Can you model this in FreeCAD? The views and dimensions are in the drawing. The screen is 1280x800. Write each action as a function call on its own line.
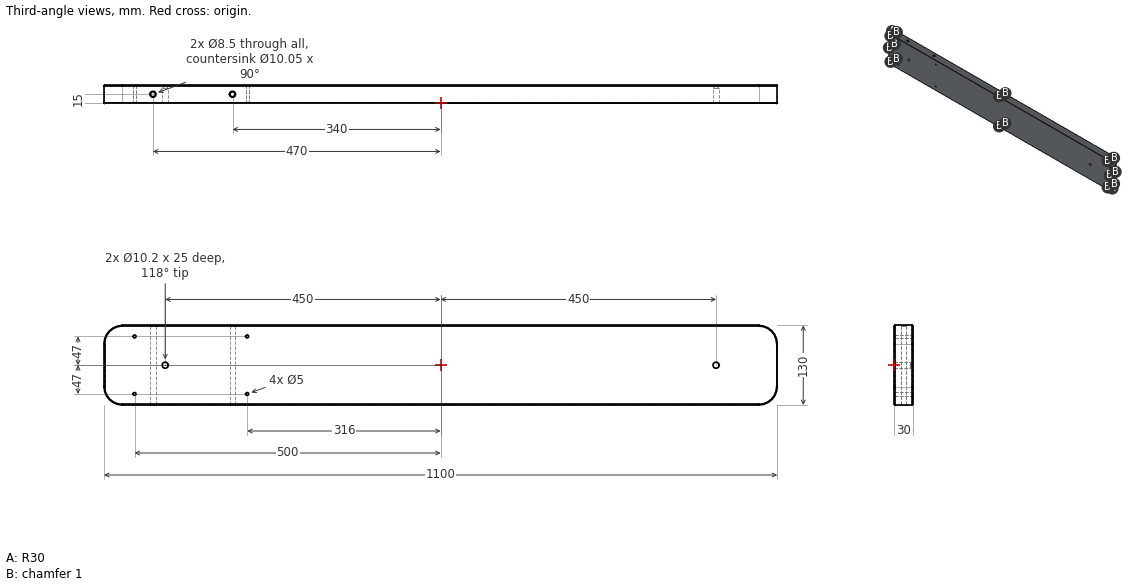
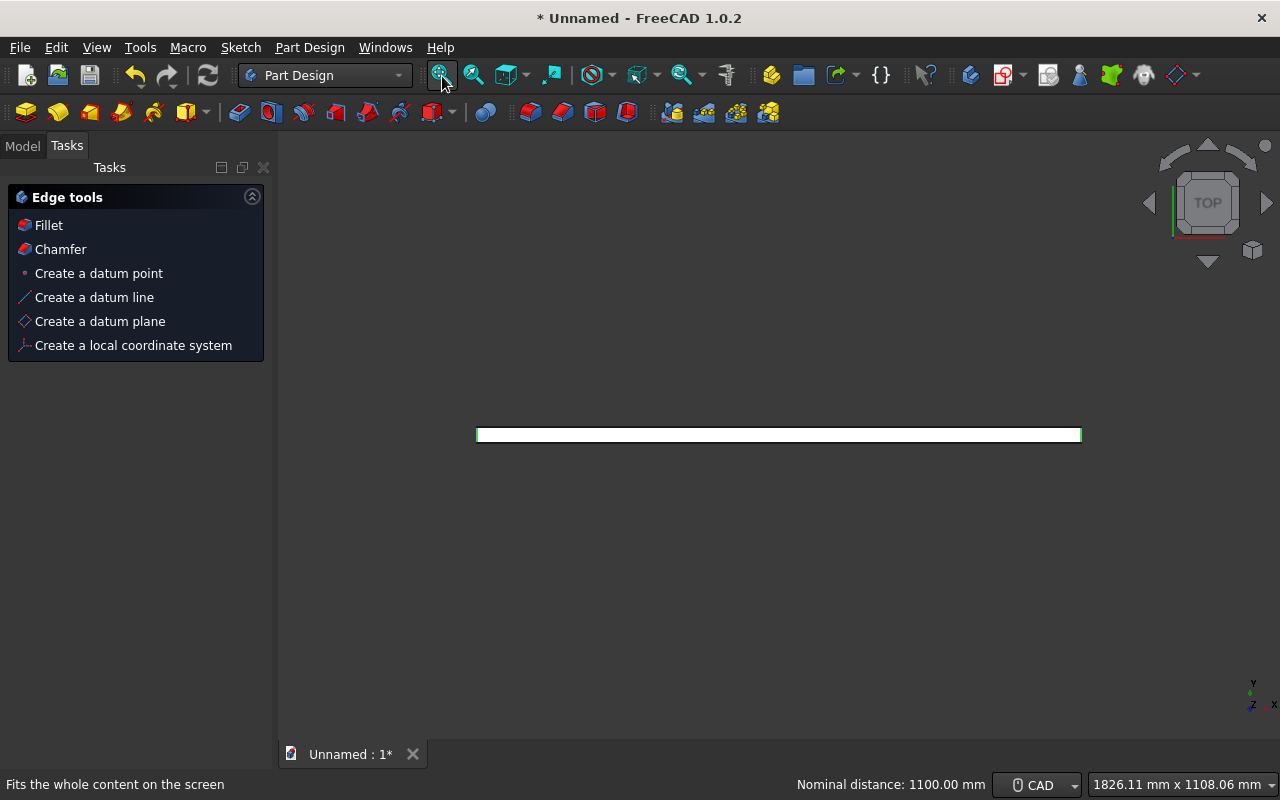
key(0)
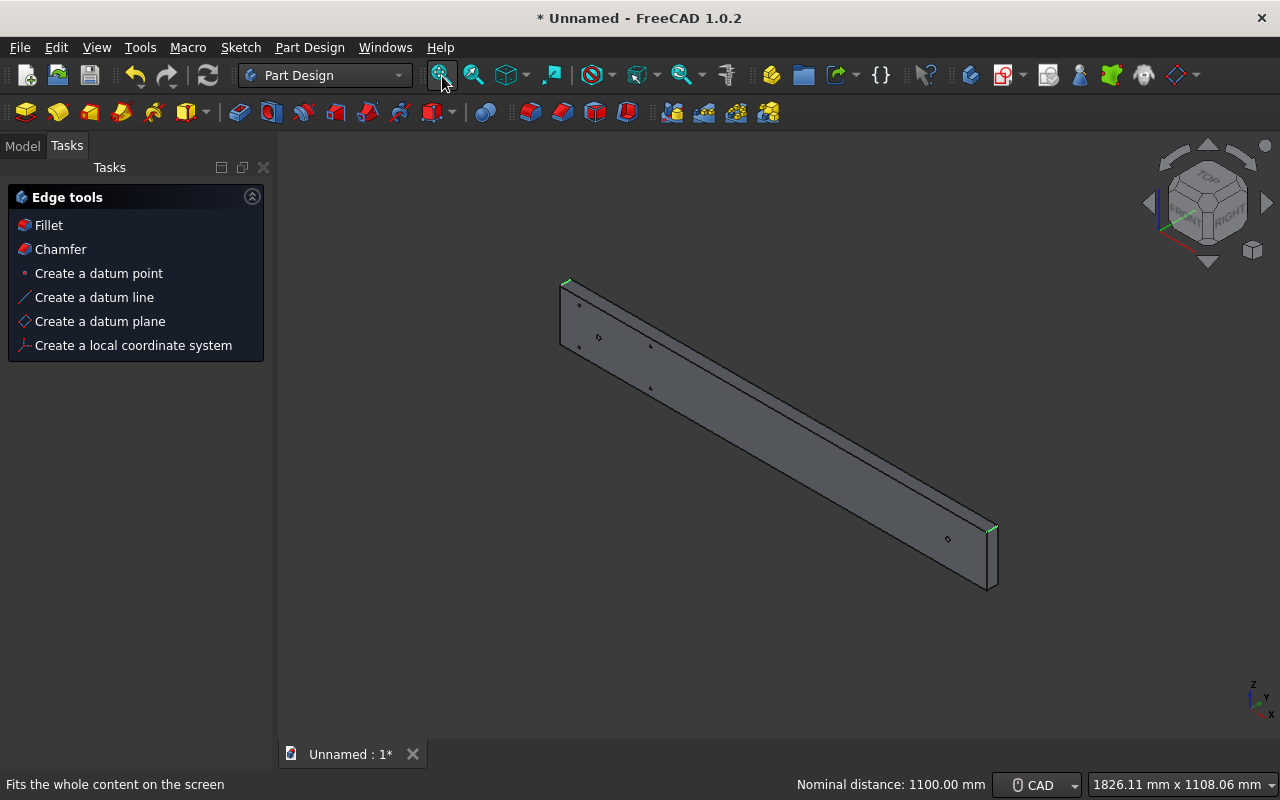
scroll(566, 340, up, 5)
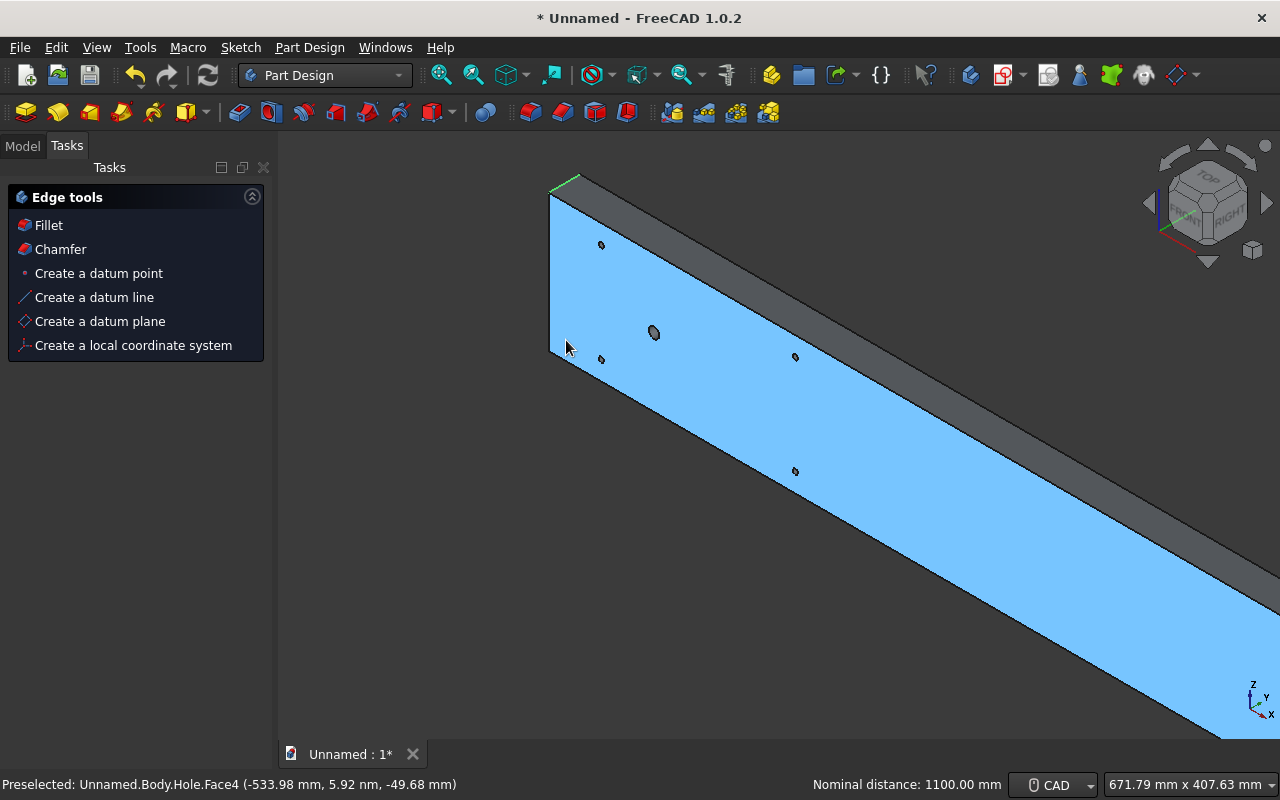
click(442, 76)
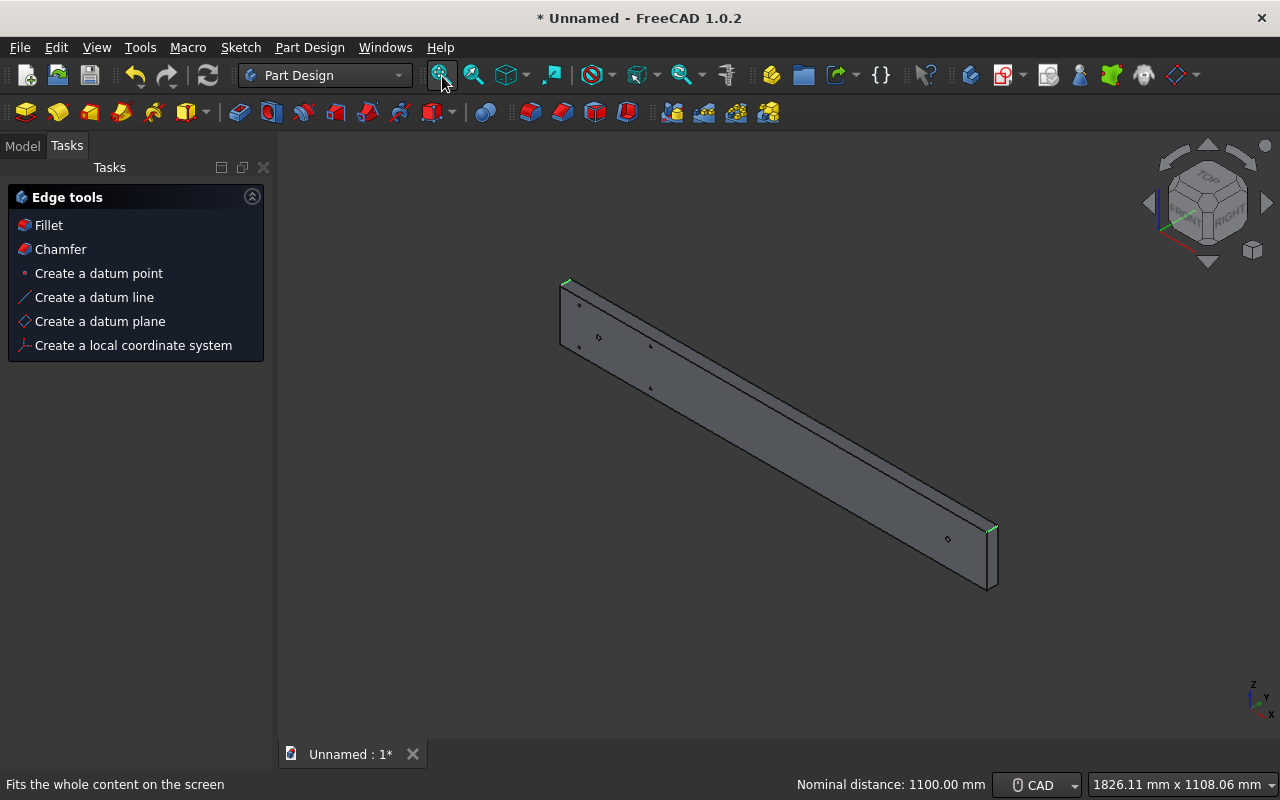
key(1)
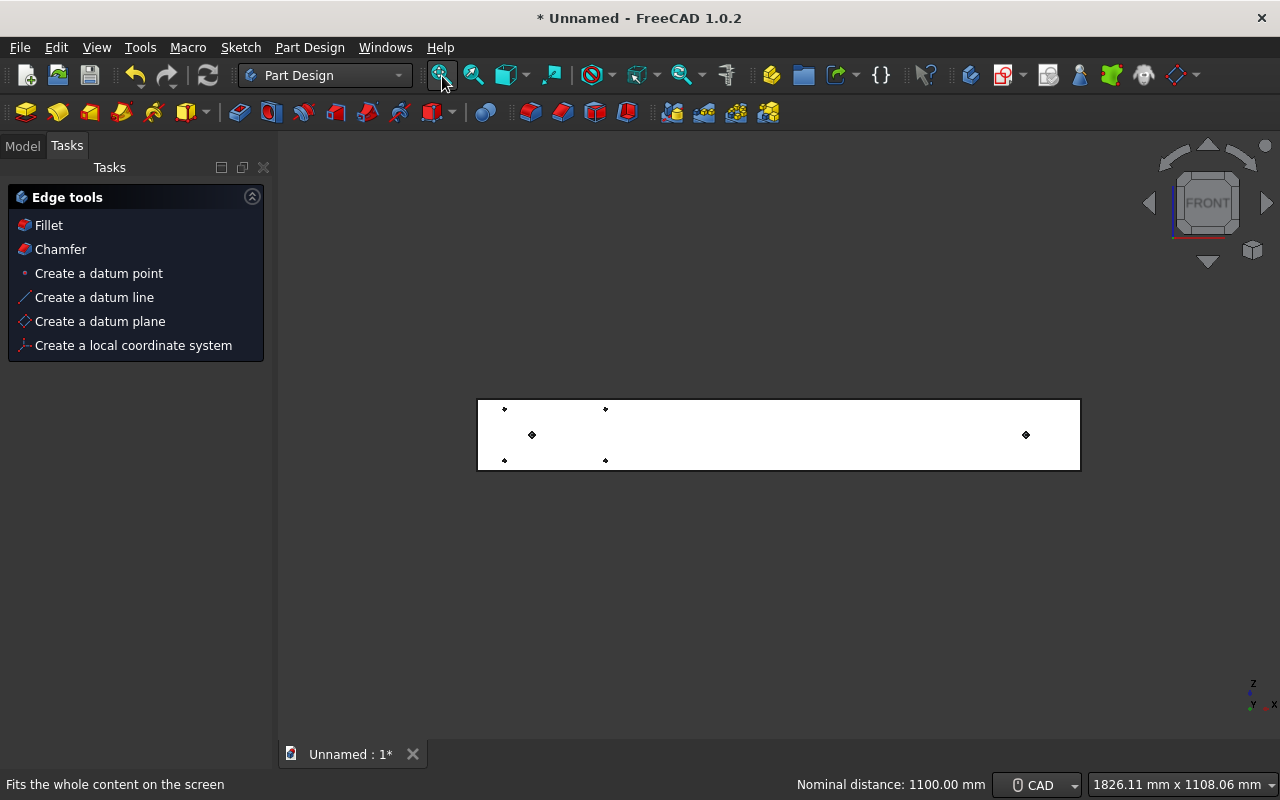
scroll(477, 470, up, 5)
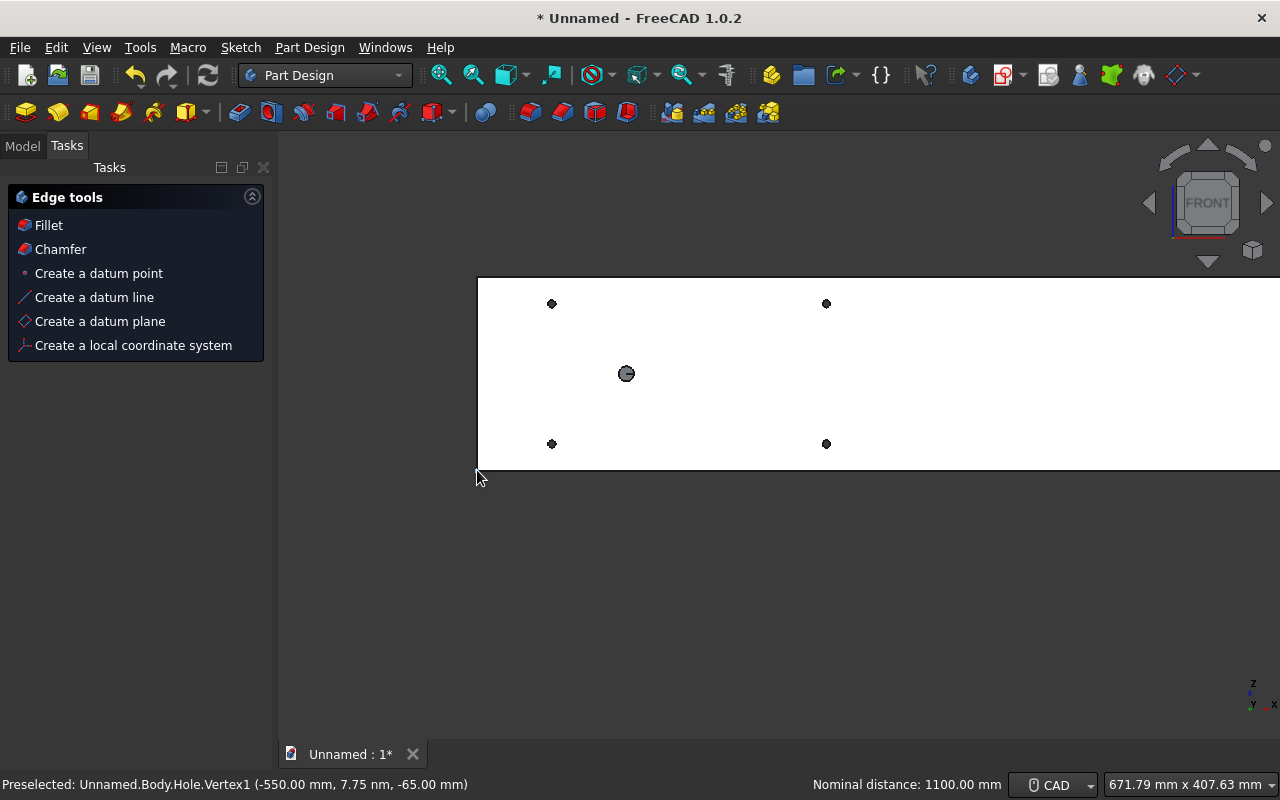
click(442, 76)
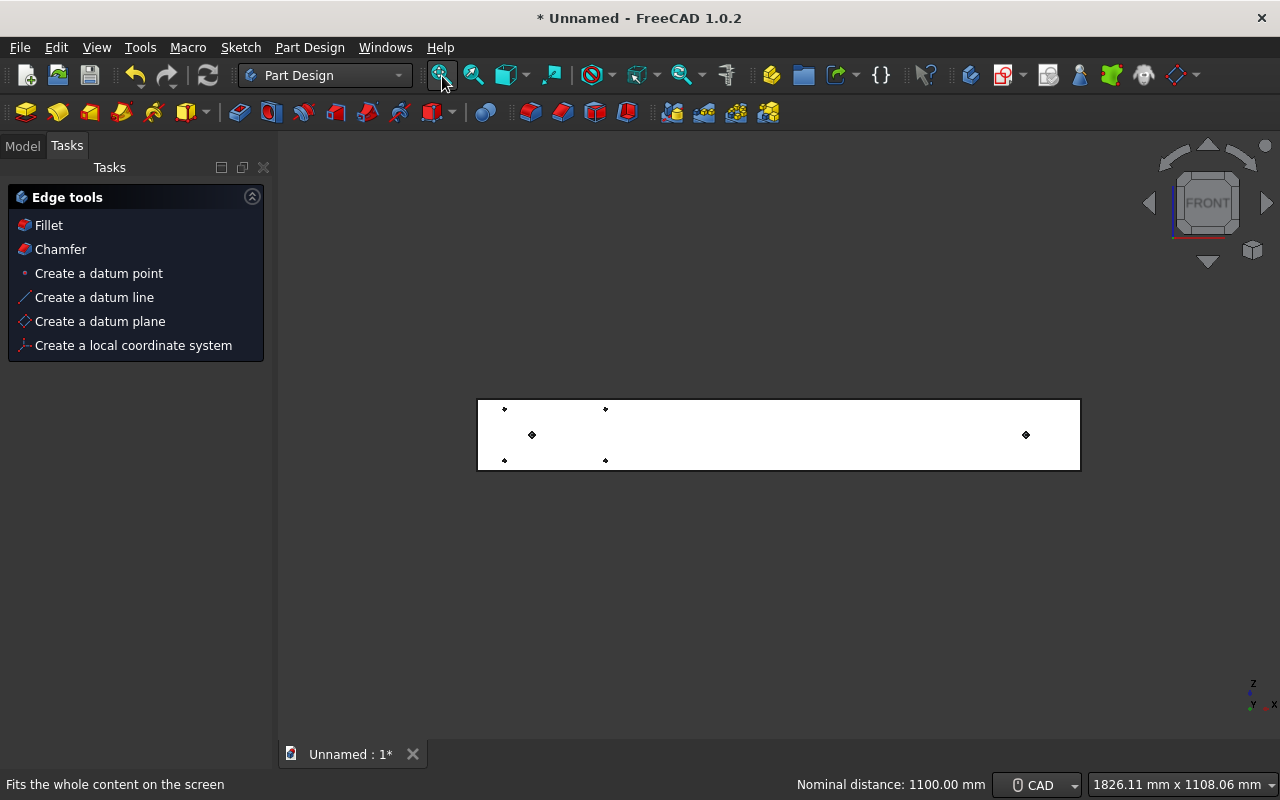
key(3)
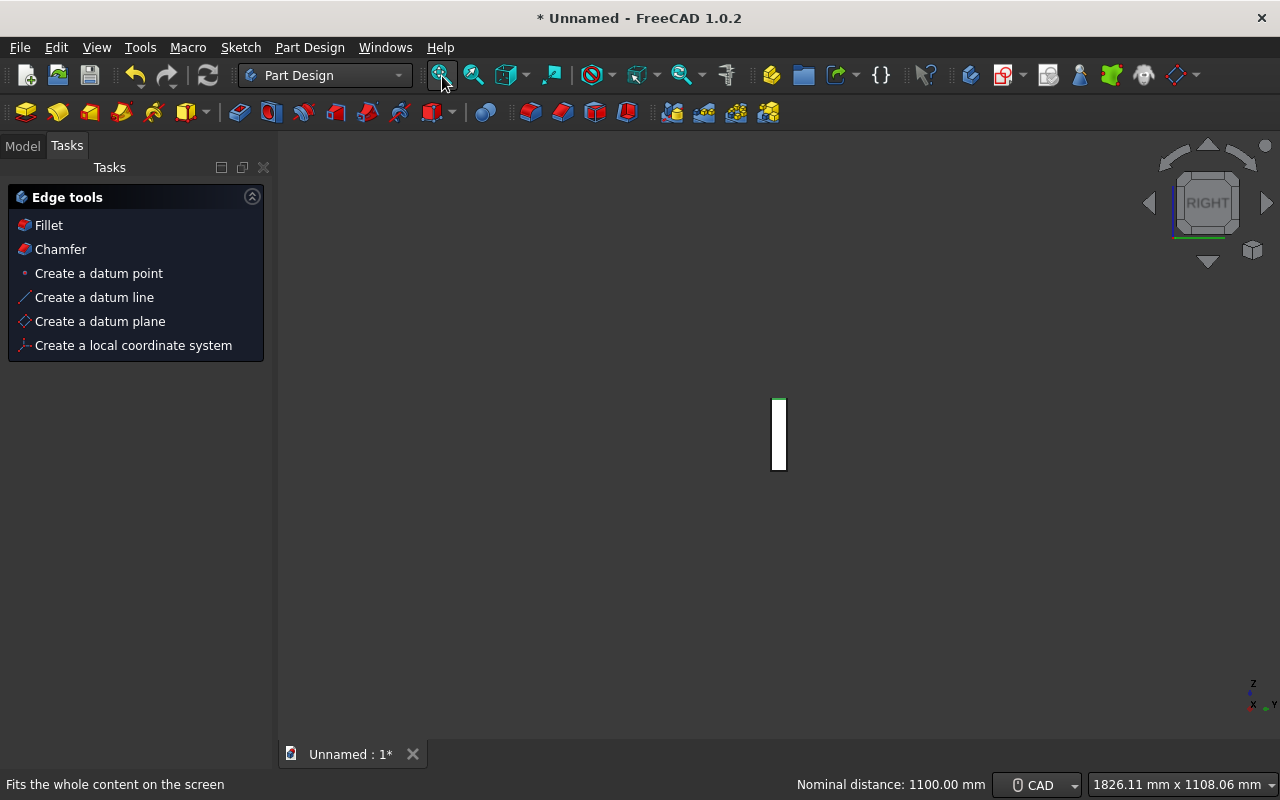
click(442, 76)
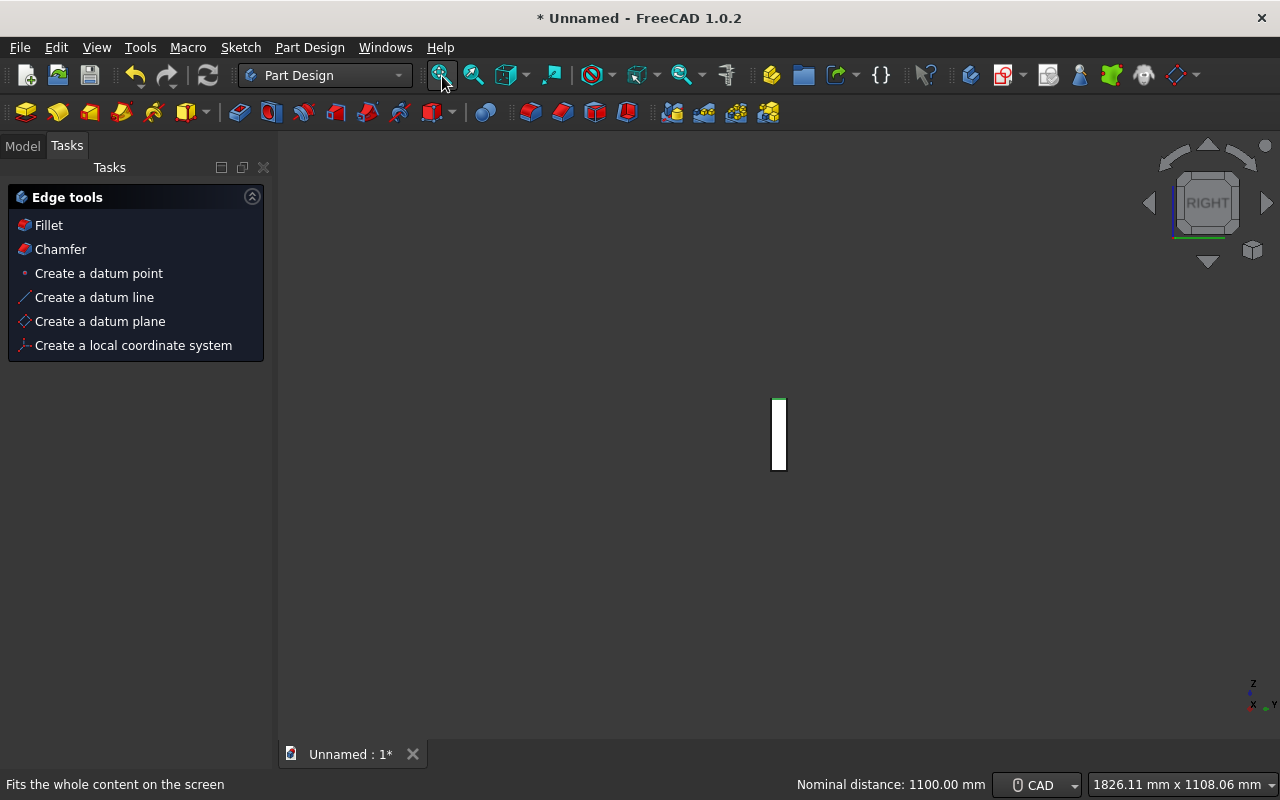
click(779, 470, ctrl)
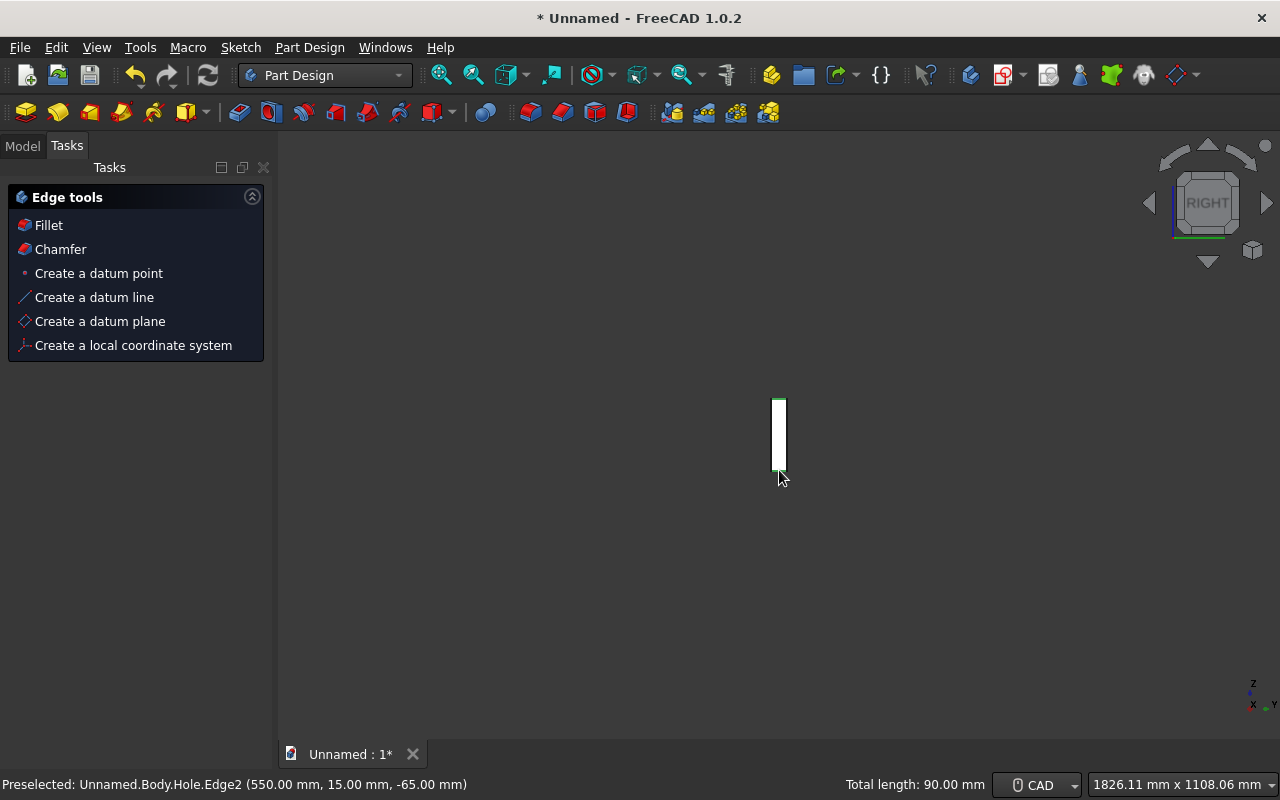
scroll(779, 470, up, 5)